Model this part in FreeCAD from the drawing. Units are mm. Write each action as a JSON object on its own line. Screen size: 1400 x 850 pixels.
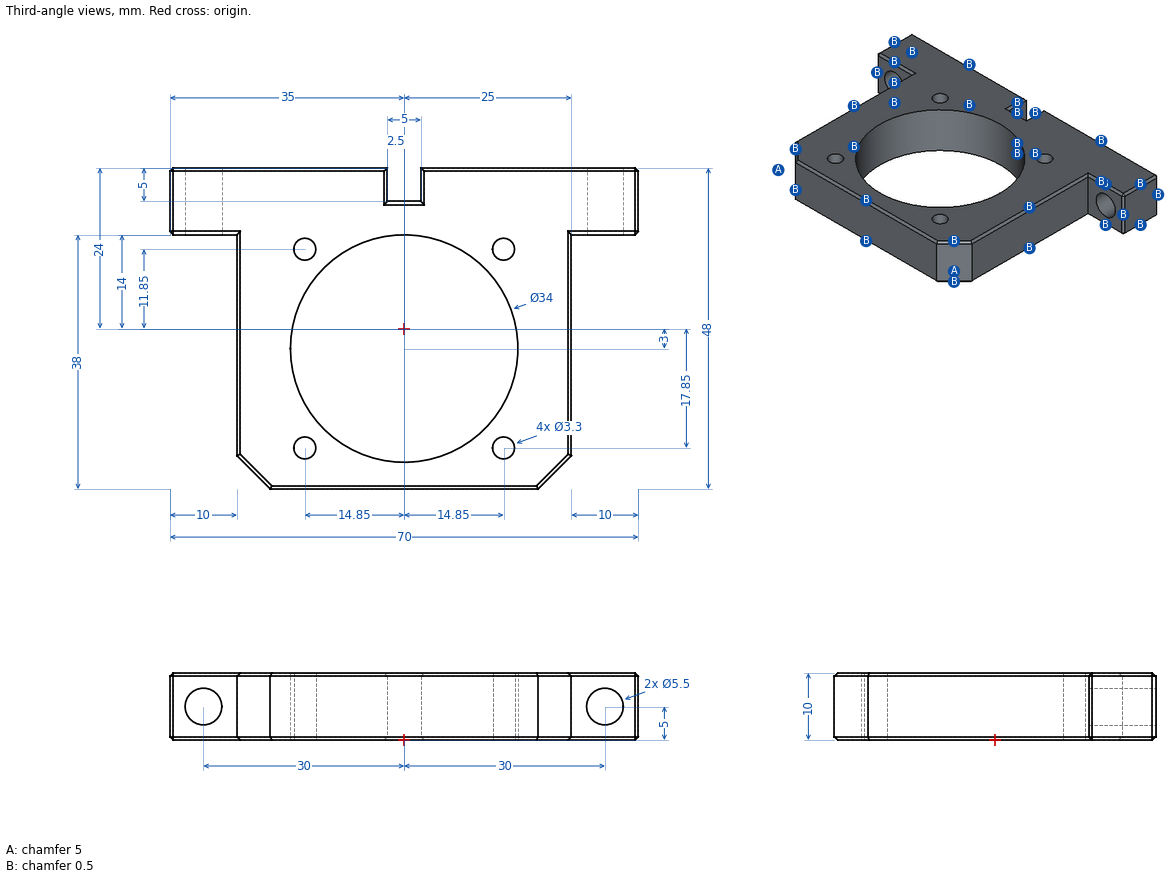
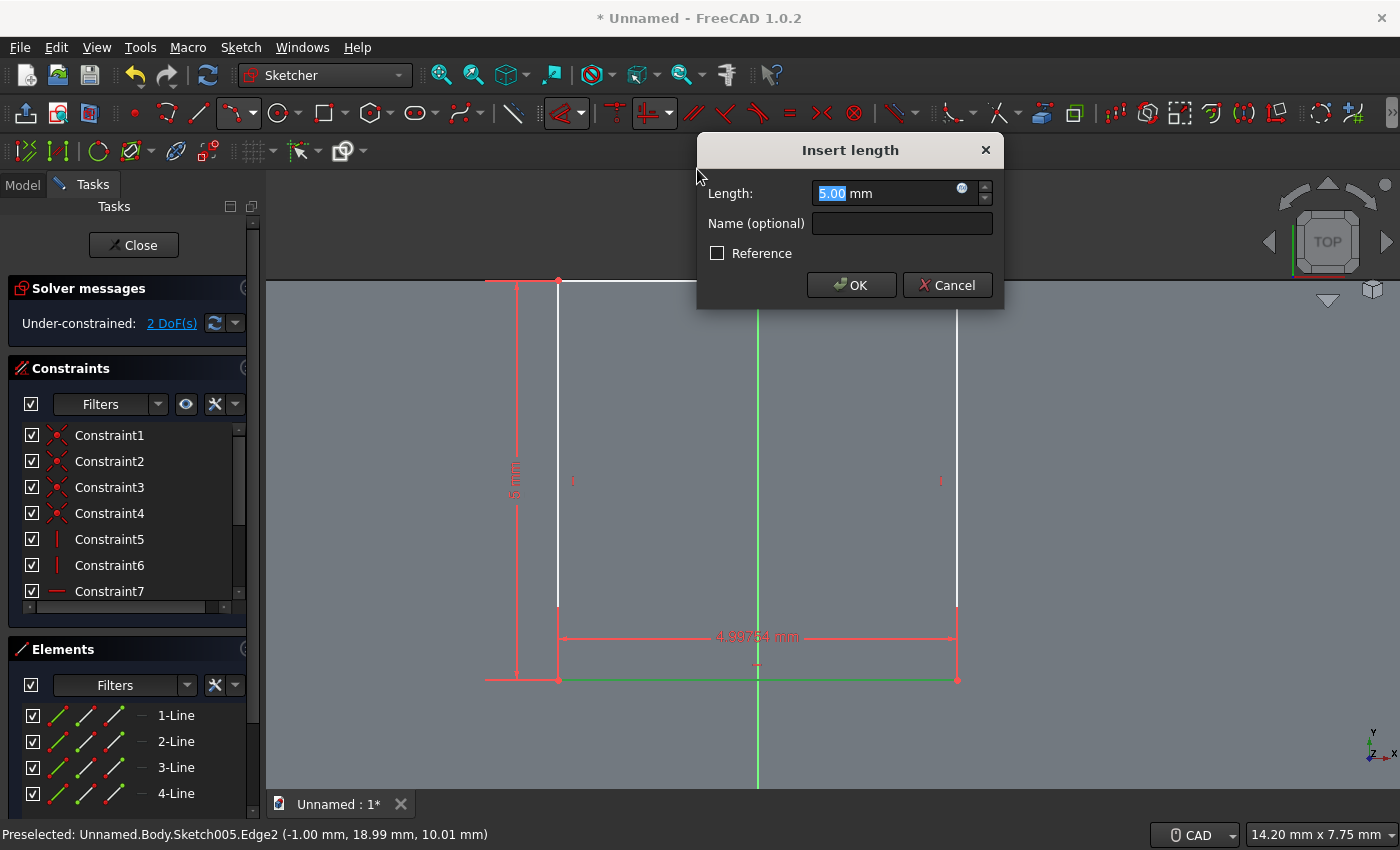
{"action": "type", "text": "5"}
{"action": "key", "text": "Return"}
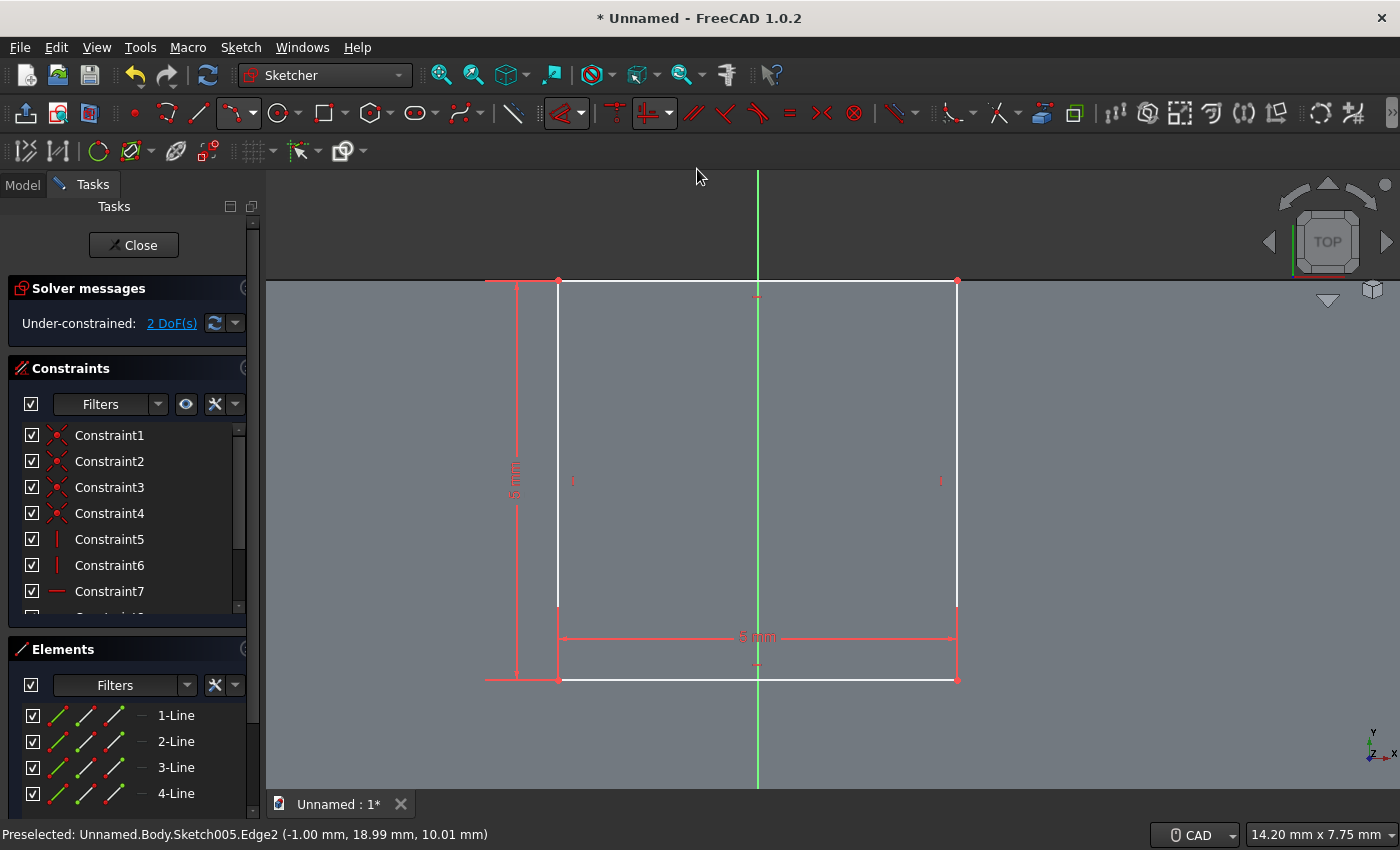
{"action": "left_click", "coordinate": [558, 281]}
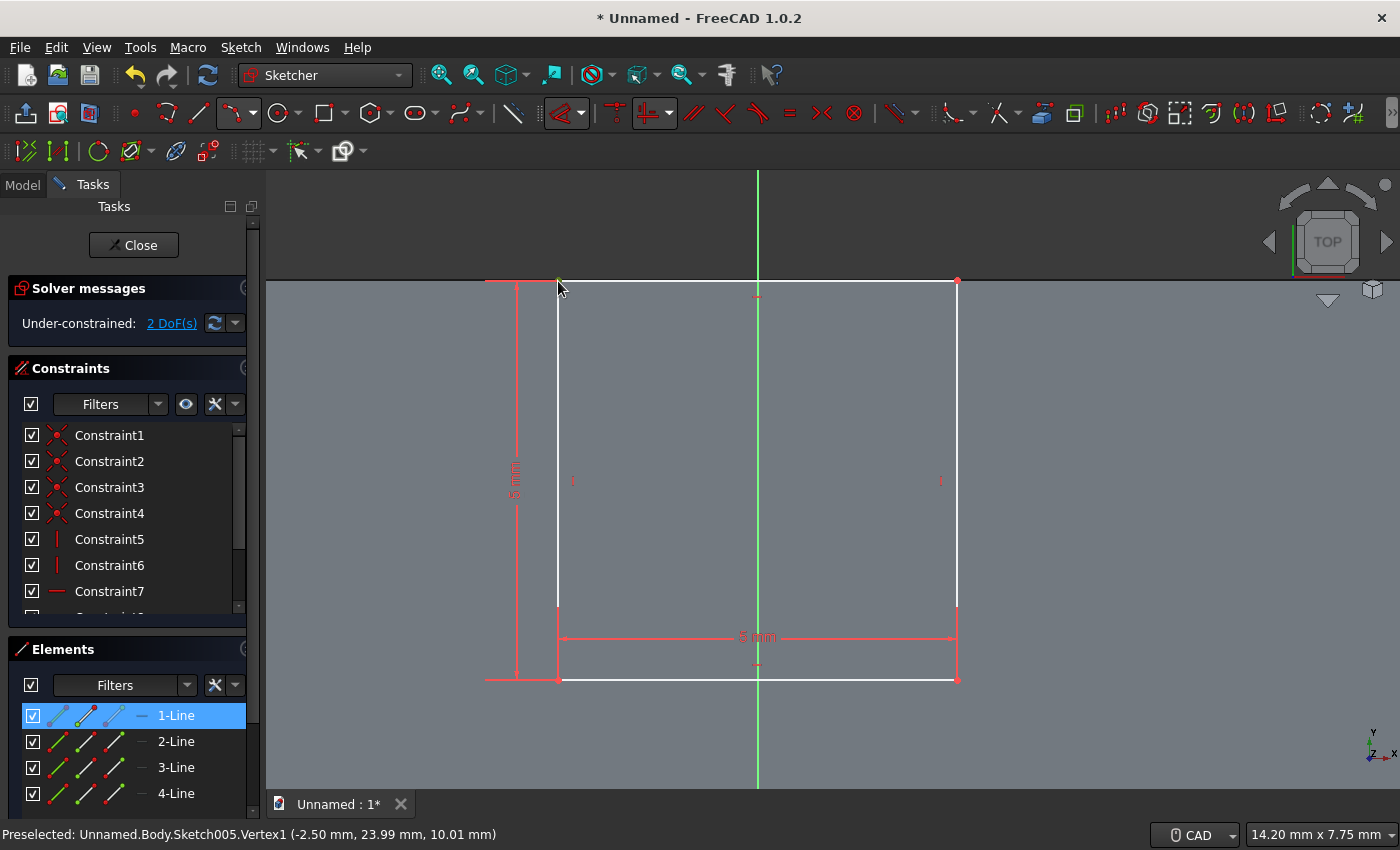
{"action": "left_click", "coordinate": [584, 114]}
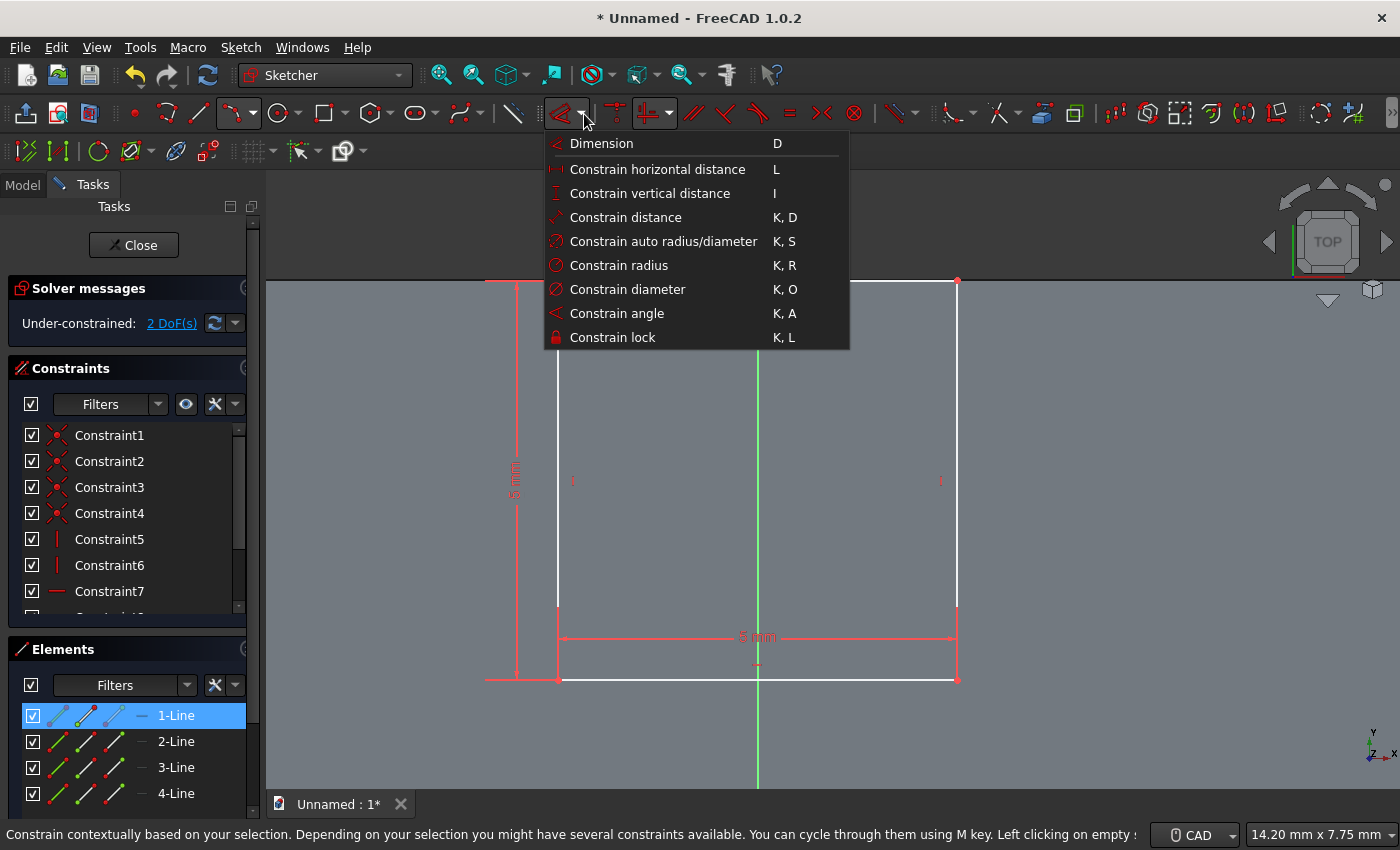
{"action": "left_click", "coordinate": [697, 193]}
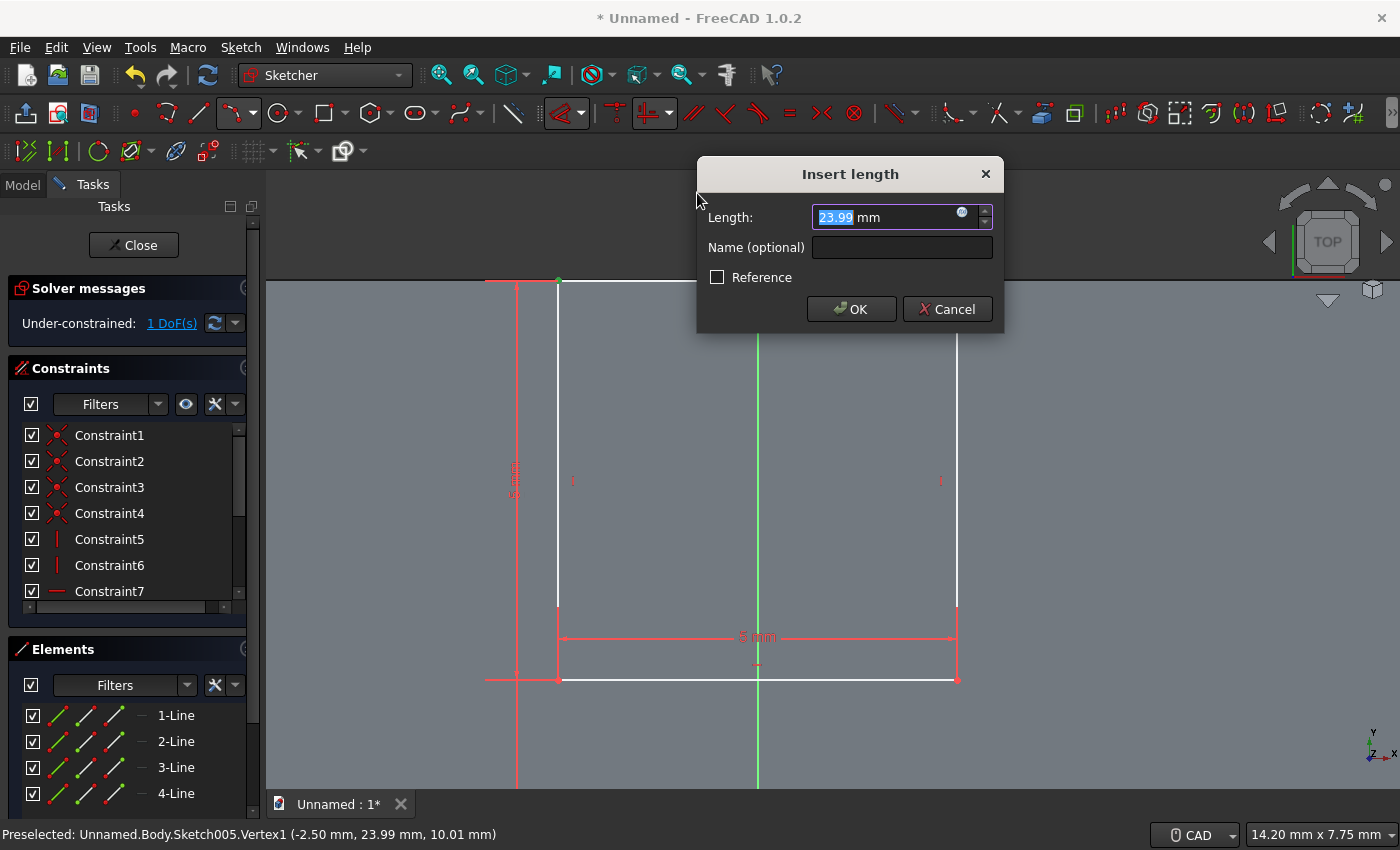
{"action": "type", "text": "24"}
{"action": "key", "text": "Return"}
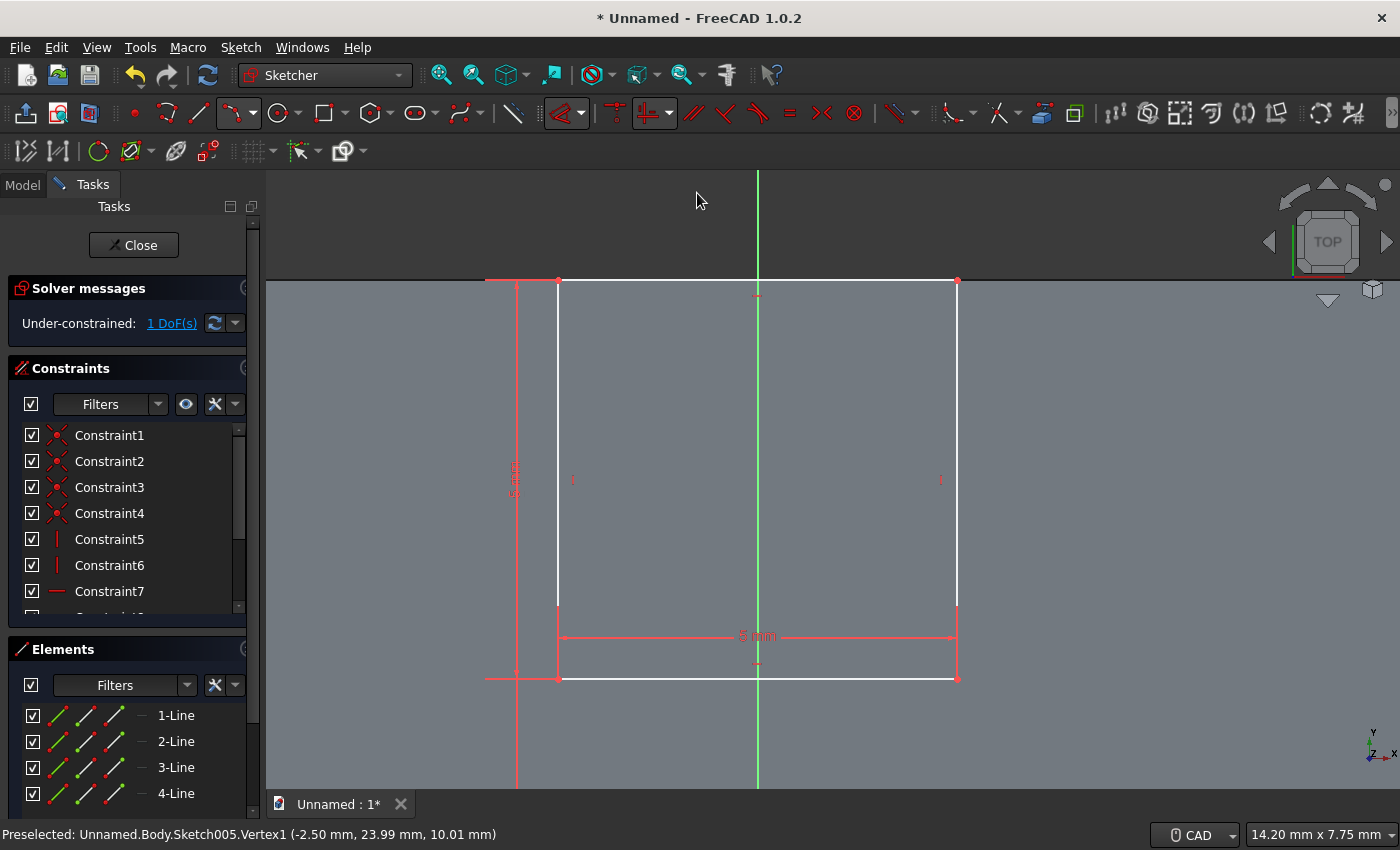
{"action": "left_click", "coordinate": [558, 280]}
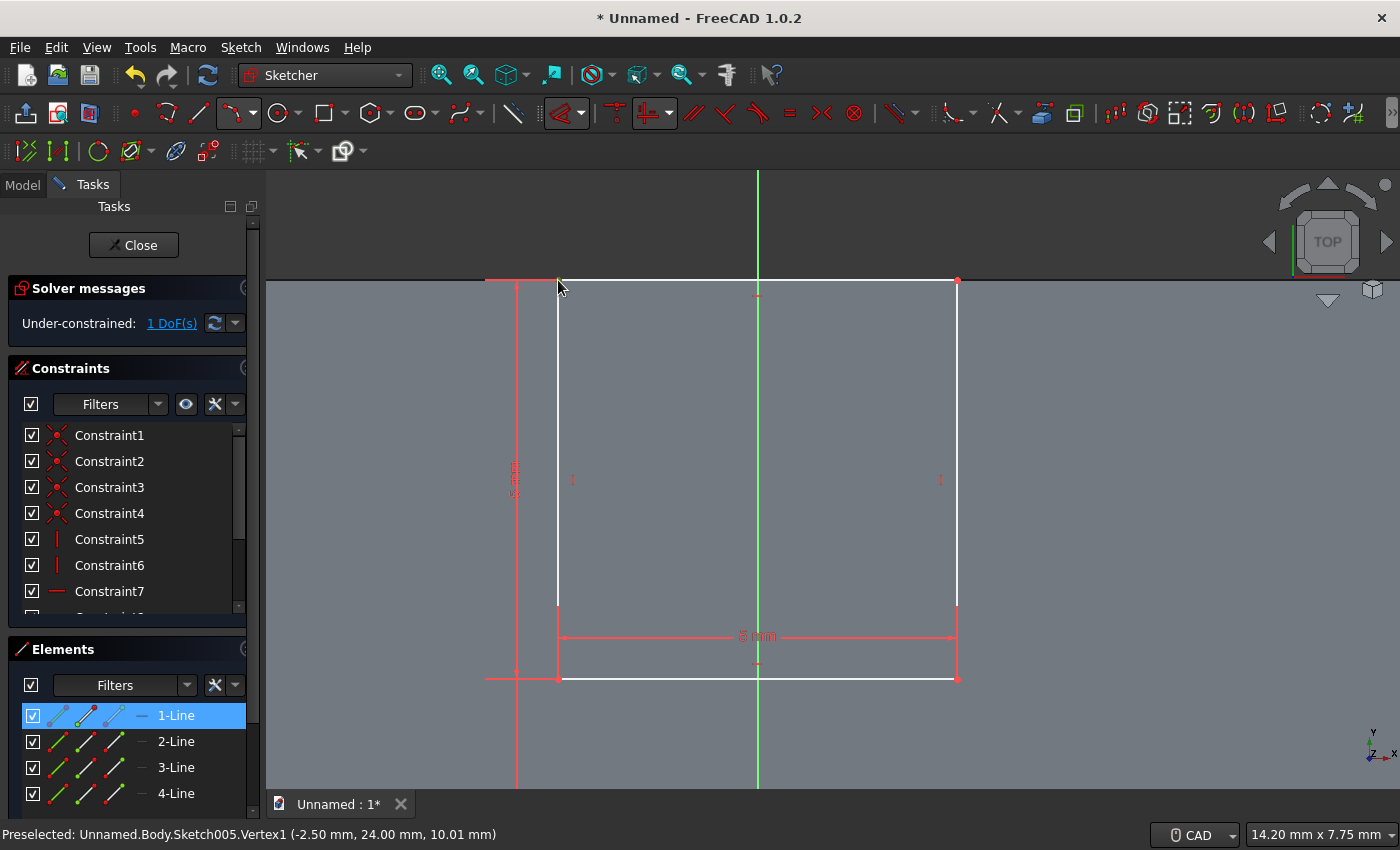
{"action": "left_click", "coordinate": [584, 114]}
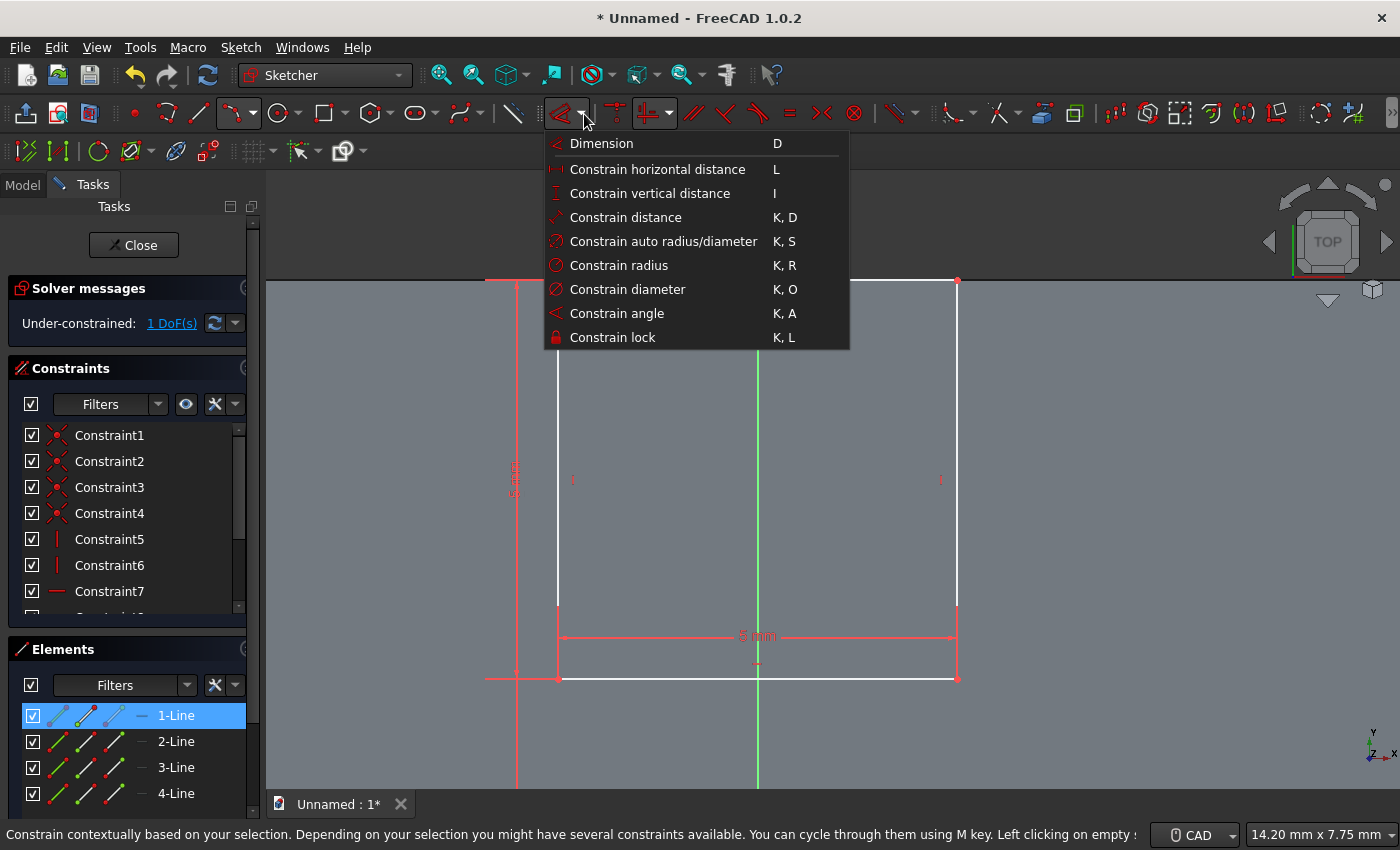
{"action": "left_click", "coordinate": [697, 169]}